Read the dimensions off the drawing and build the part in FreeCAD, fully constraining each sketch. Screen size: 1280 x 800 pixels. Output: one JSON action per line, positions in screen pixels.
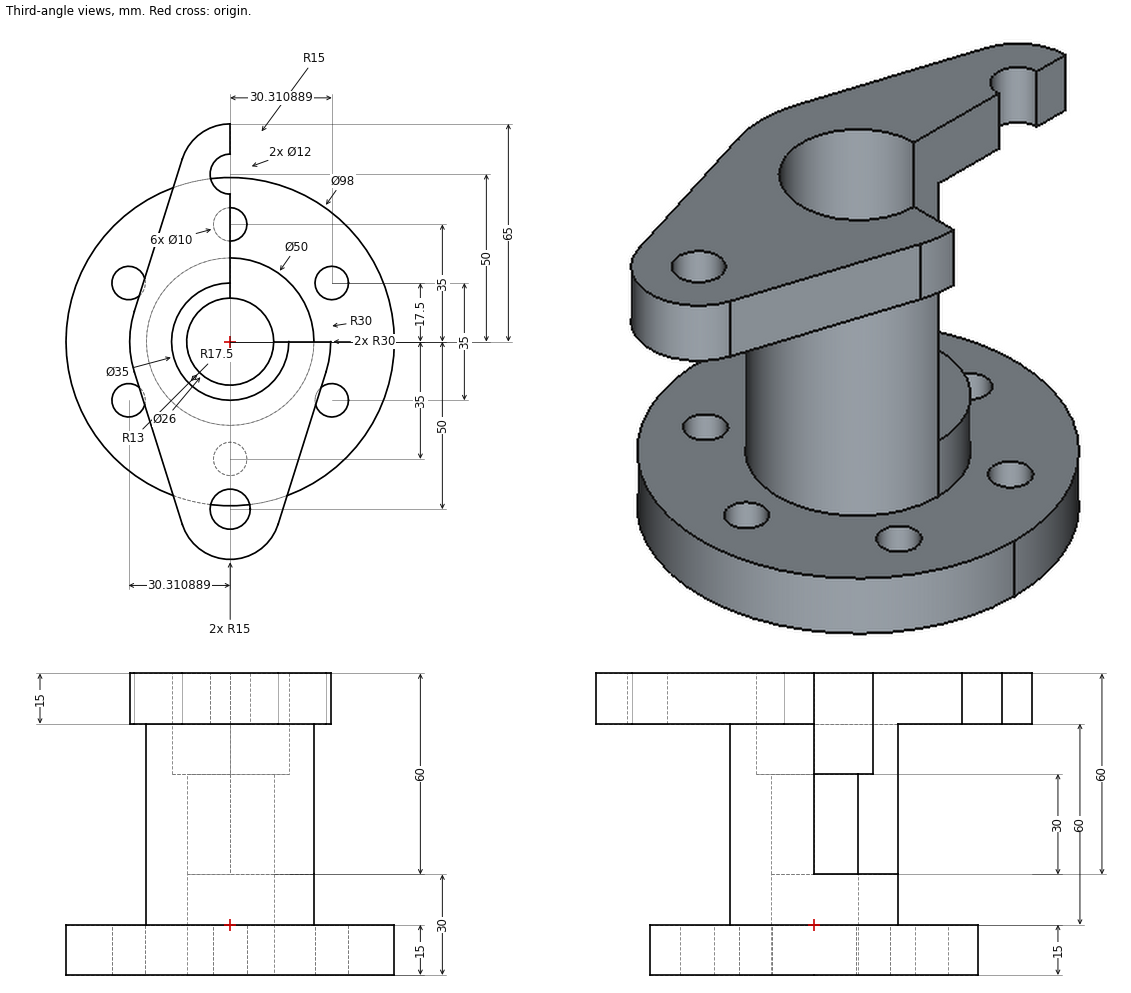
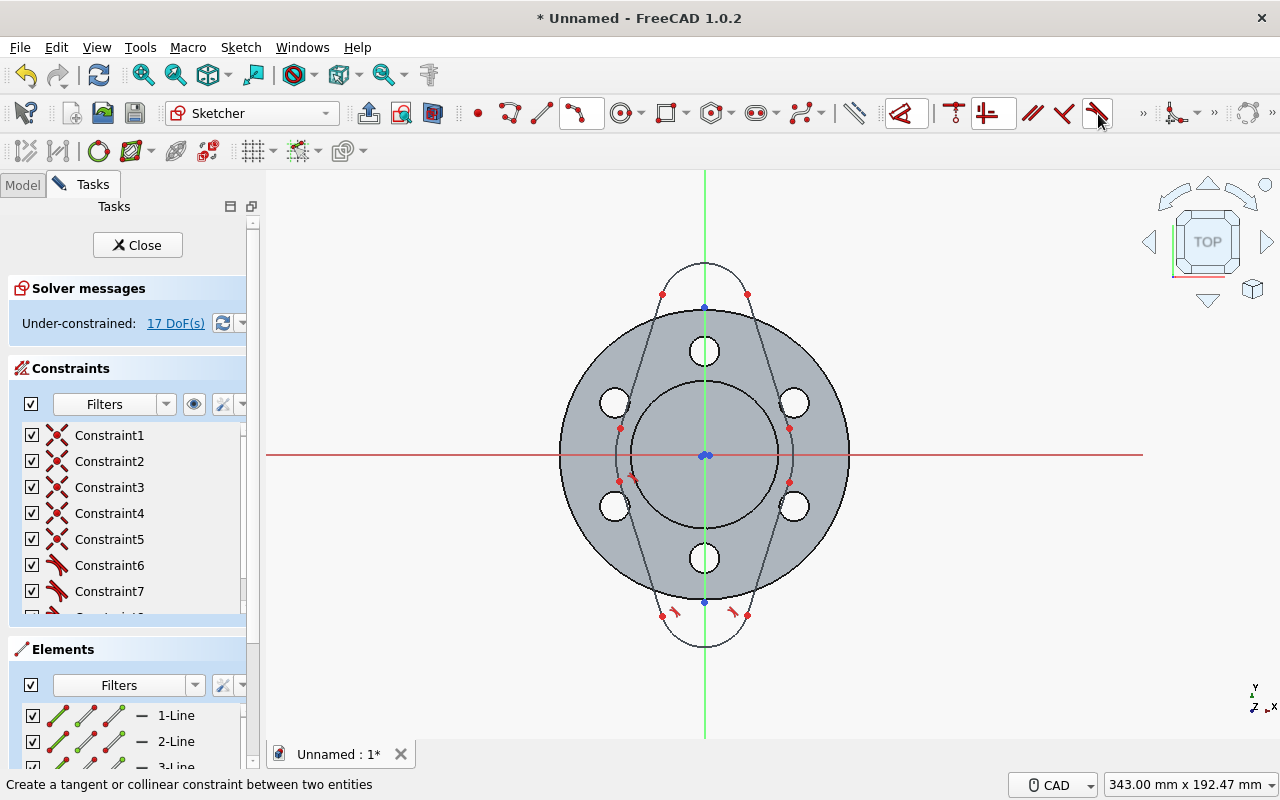
{"action": "left_click", "coordinate": [760, 576]}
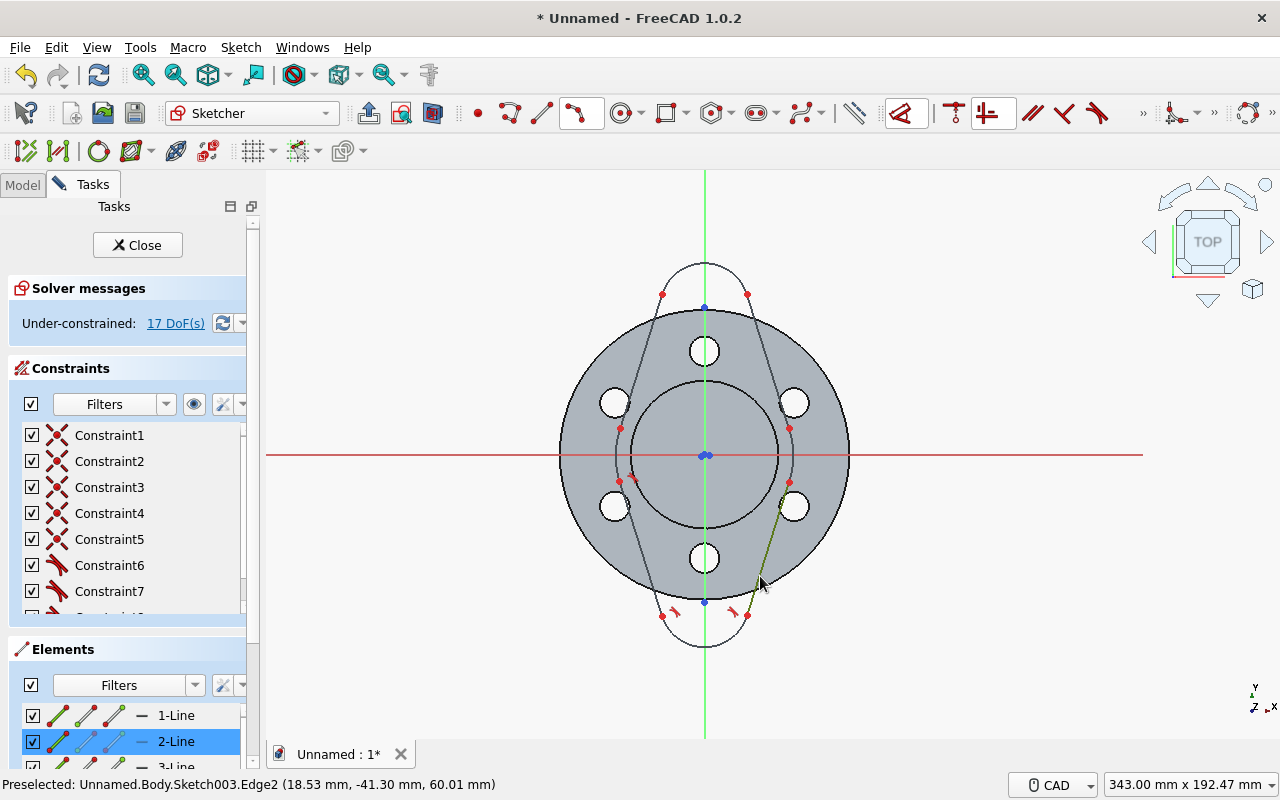
{"action": "left_click", "coordinate": [793, 466]}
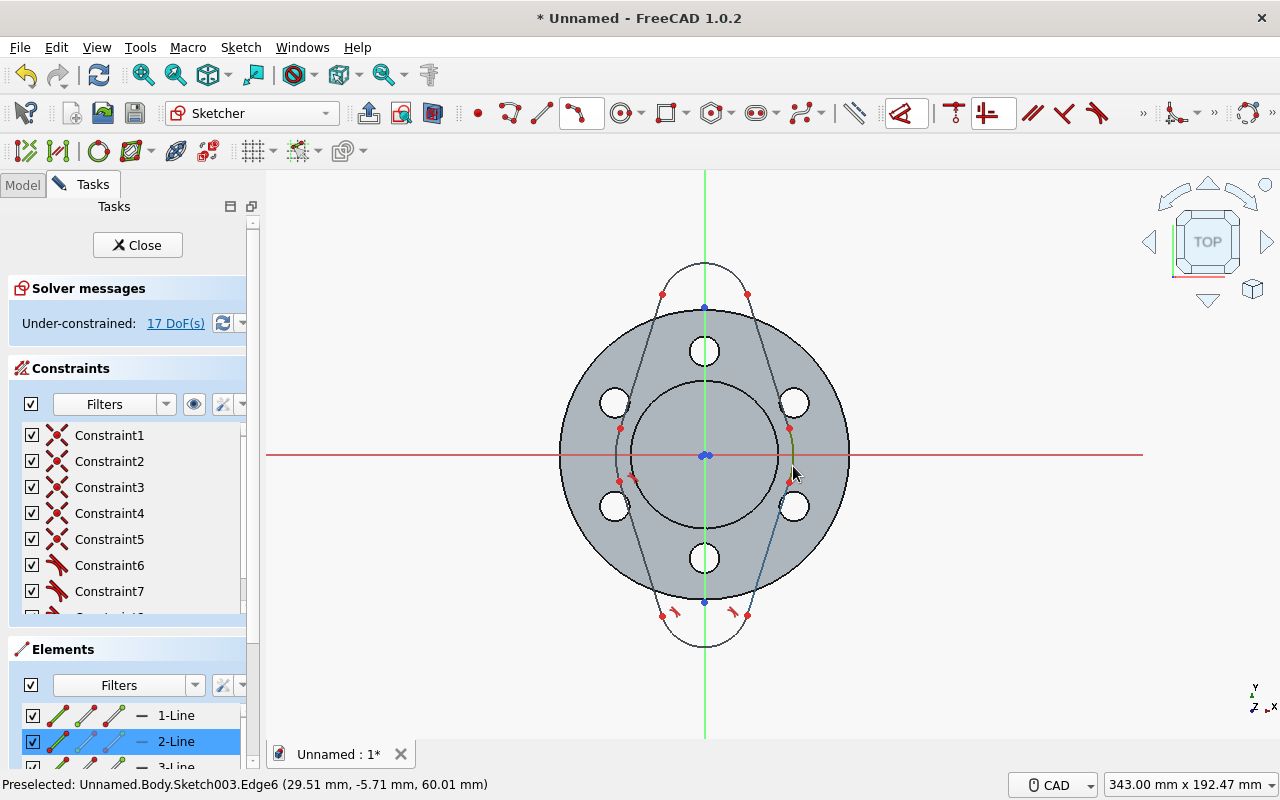
{"action": "key", "text": "t"}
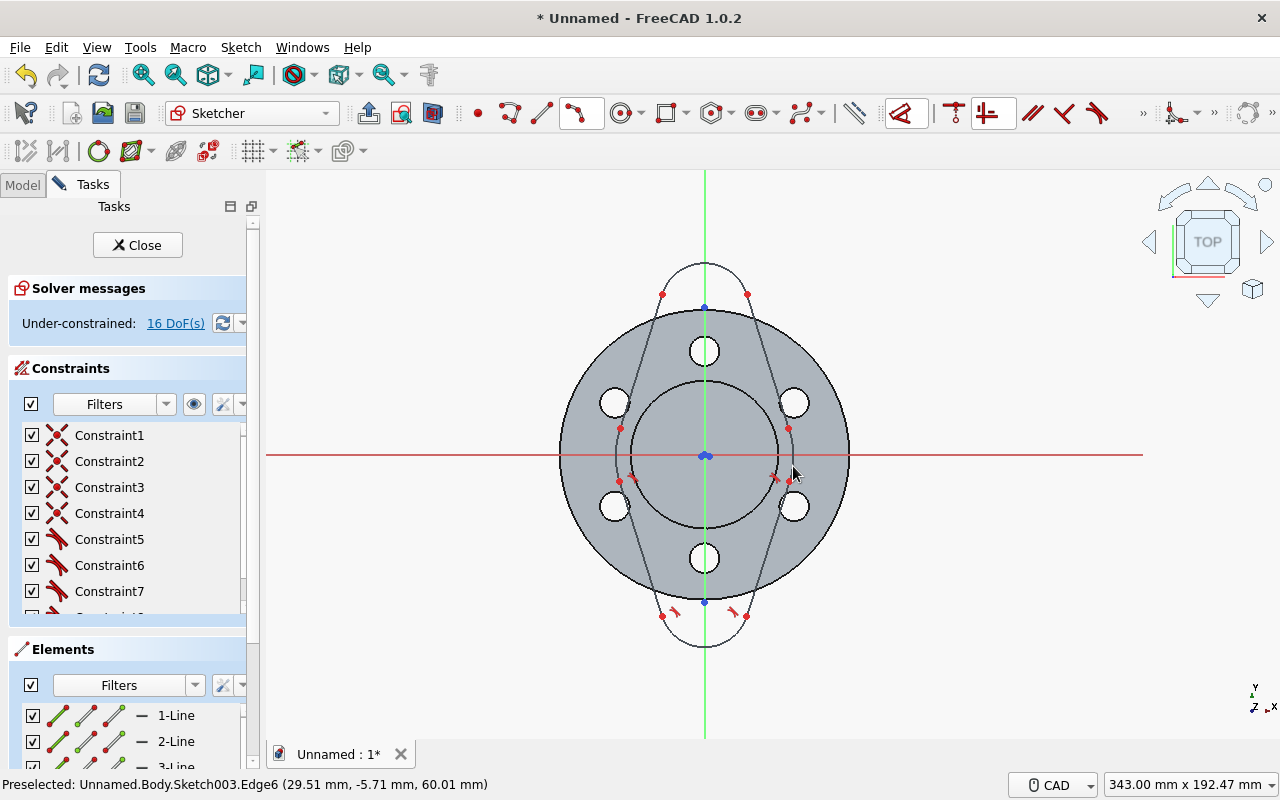
{"action": "left_click", "coordinate": [776, 389]}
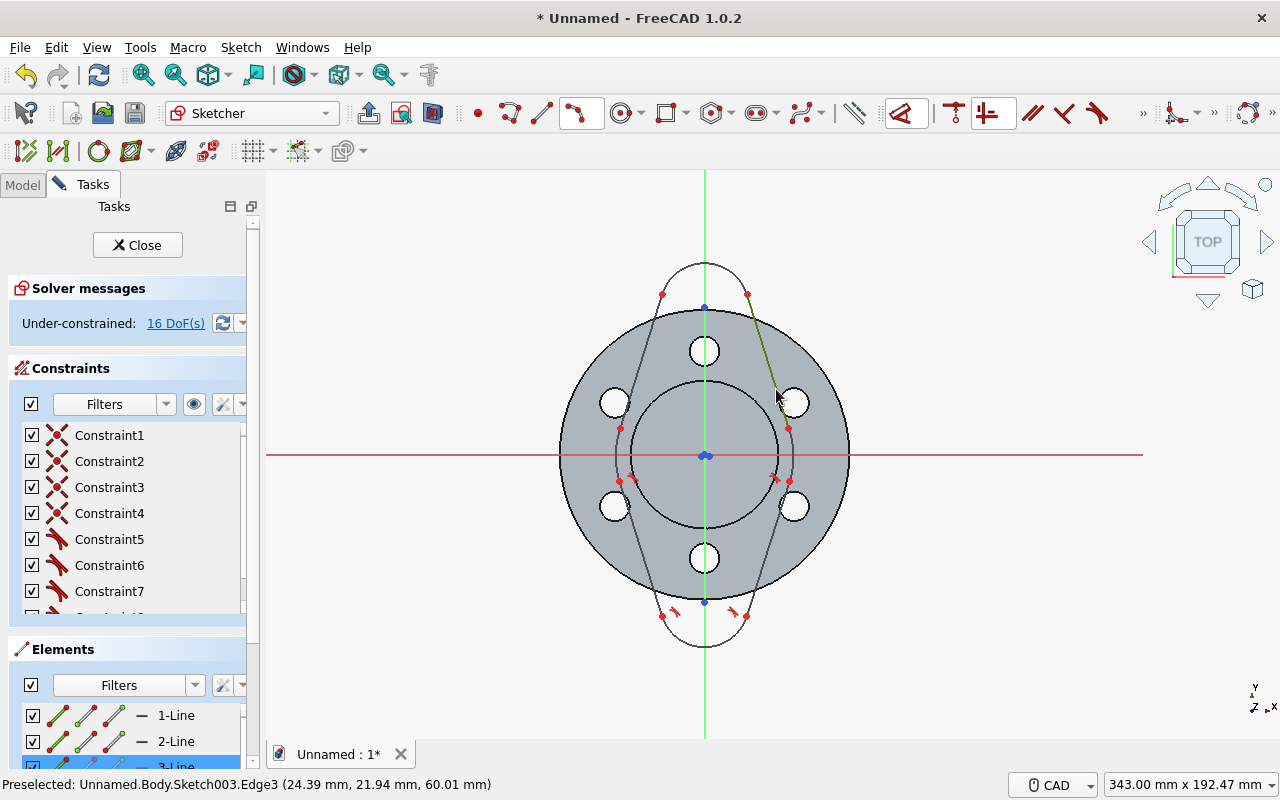
{"action": "left_click", "coordinate": [793, 466]}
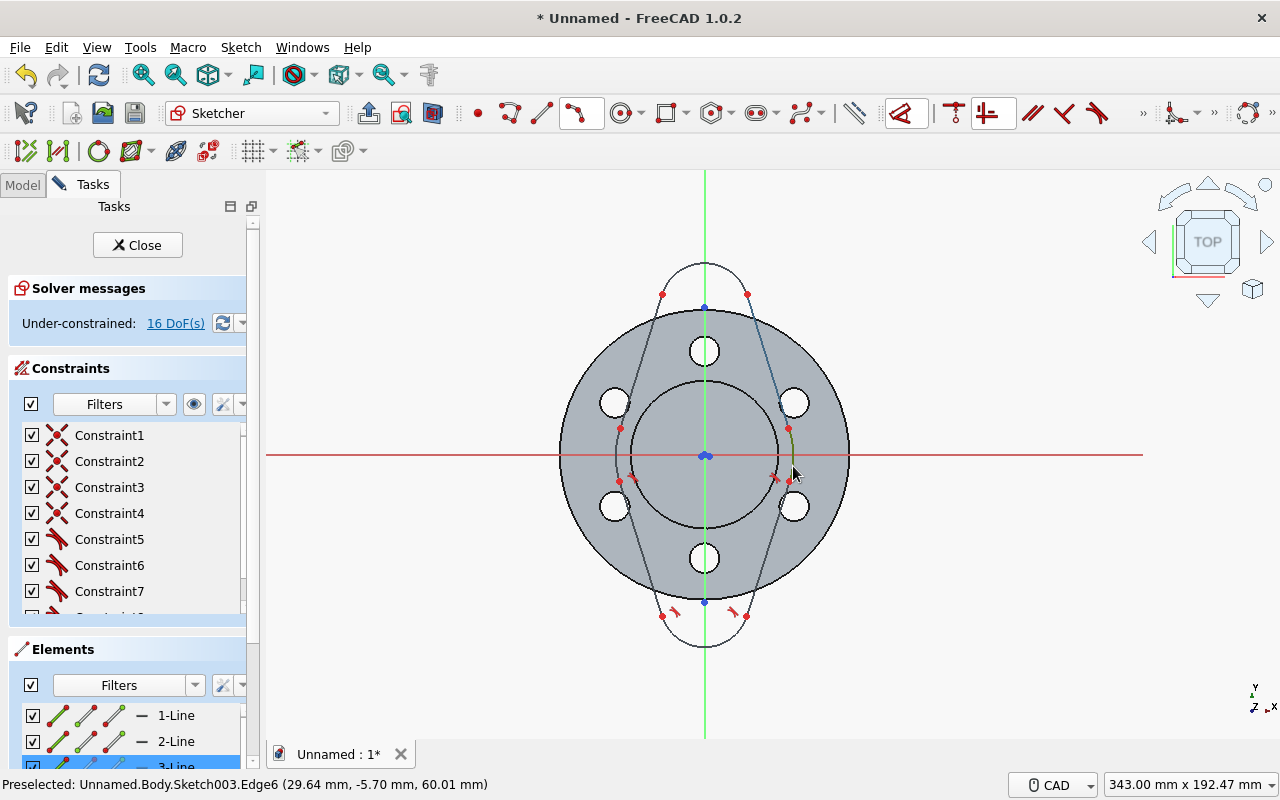
{"action": "left_click", "coordinate": [1098, 114]}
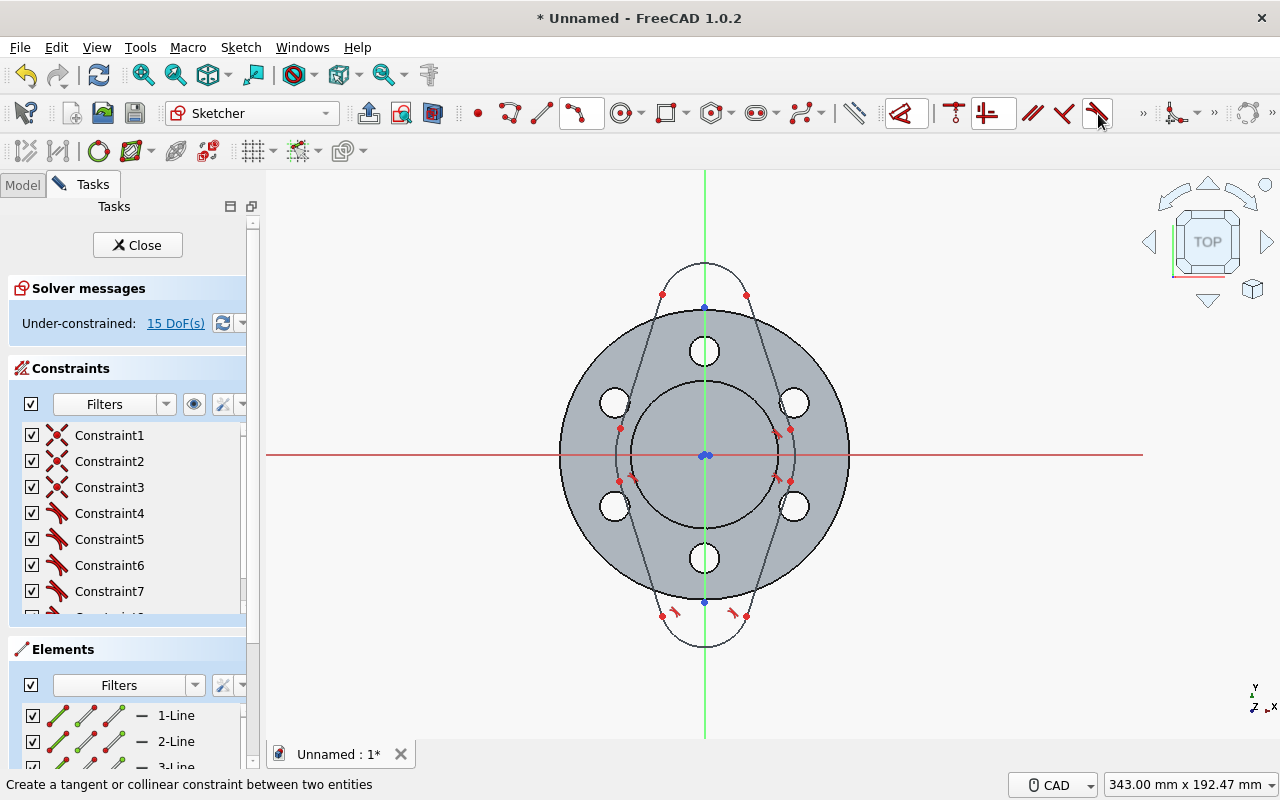
{"action": "left_click", "coordinate": [778, 389]}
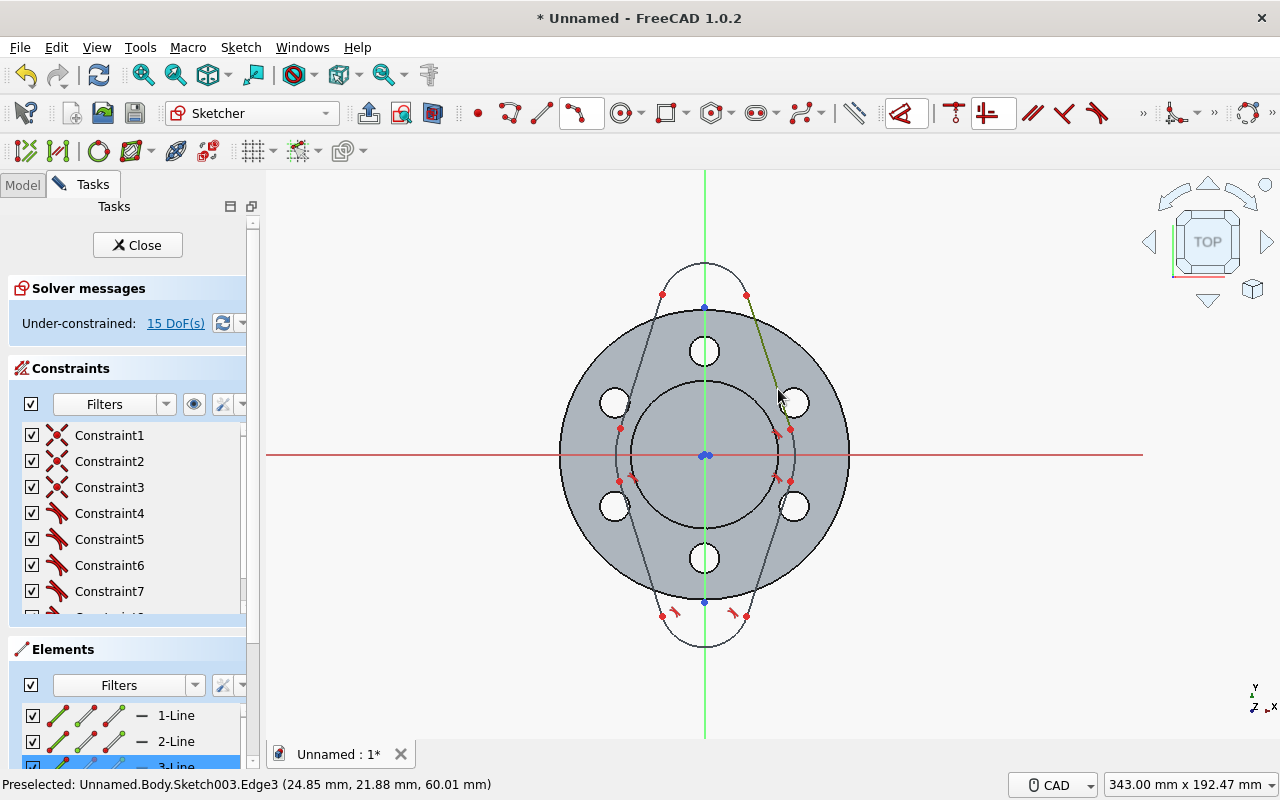
{"action": "left_click", "coordinate": [726, 269]}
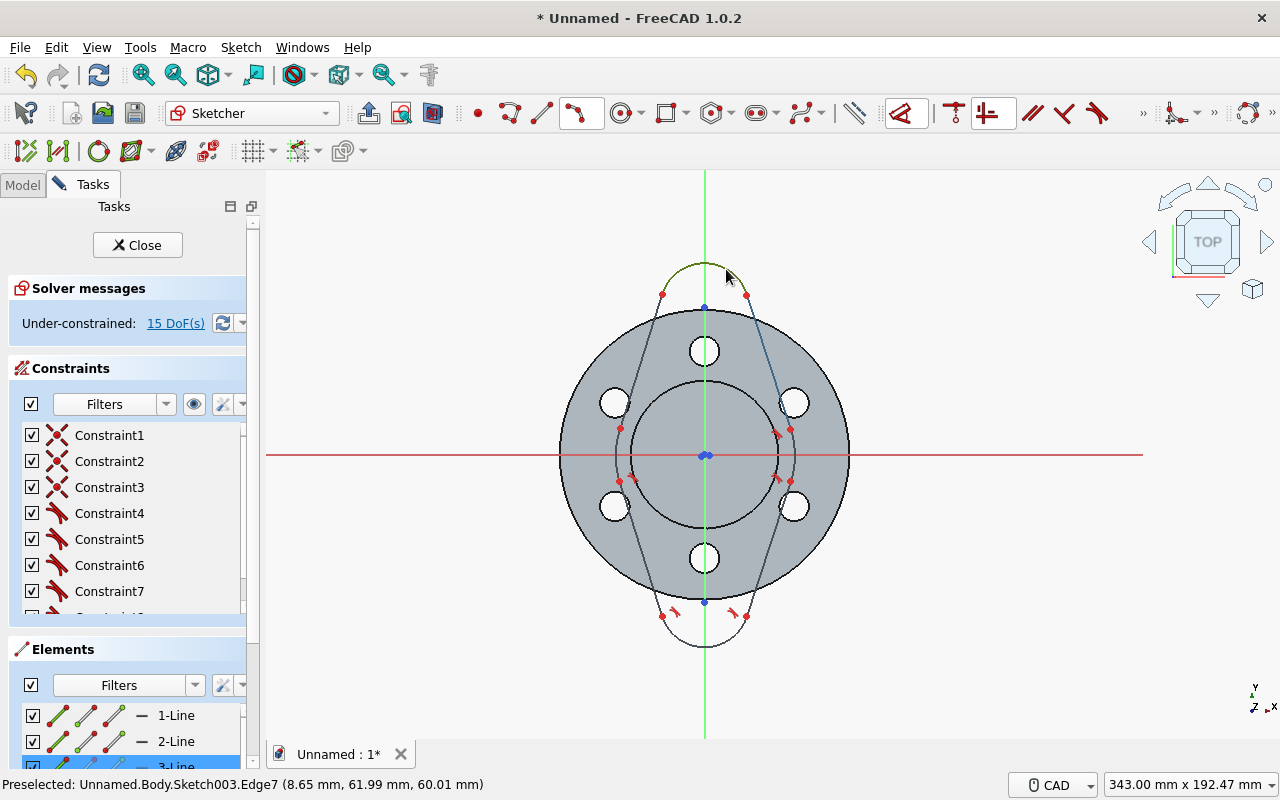
{"action": "left_click", "coordinate": [1098, 114]}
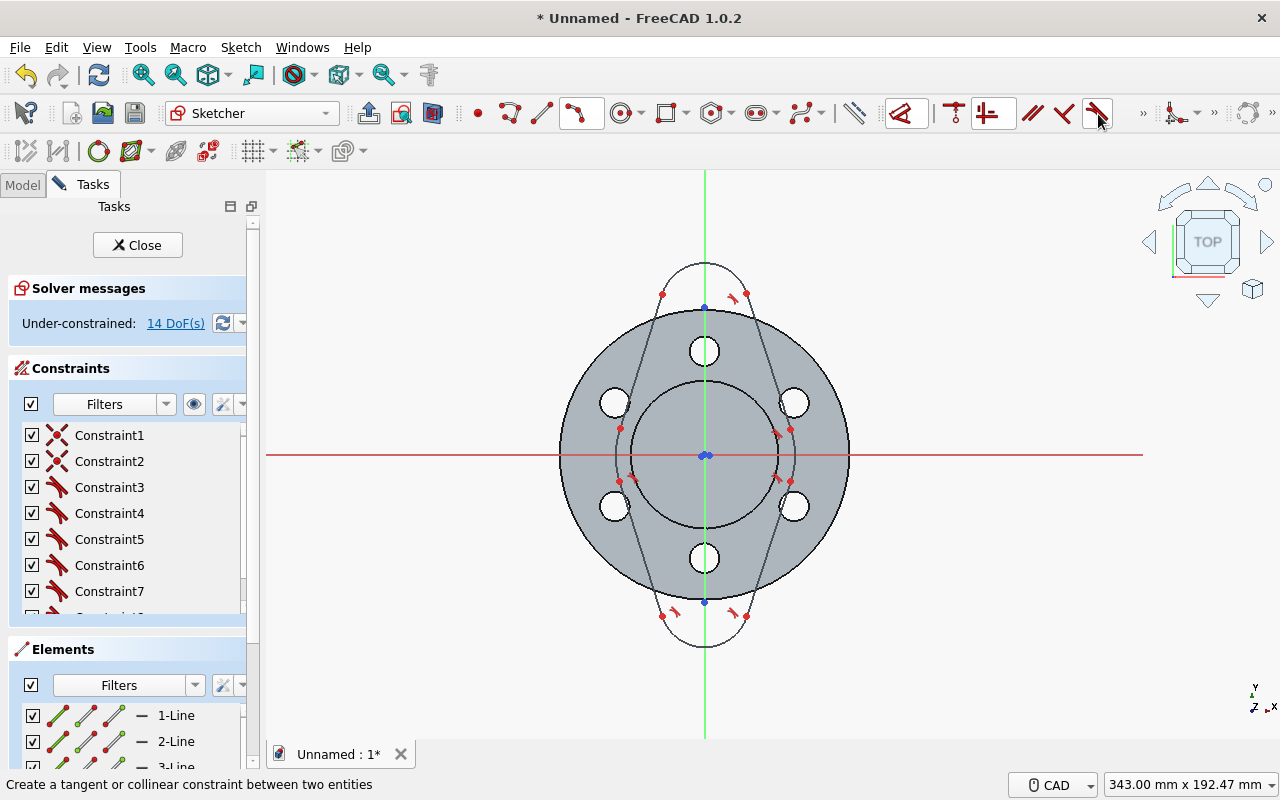
{"action": "left_click", "coordinate": [649, 335]}